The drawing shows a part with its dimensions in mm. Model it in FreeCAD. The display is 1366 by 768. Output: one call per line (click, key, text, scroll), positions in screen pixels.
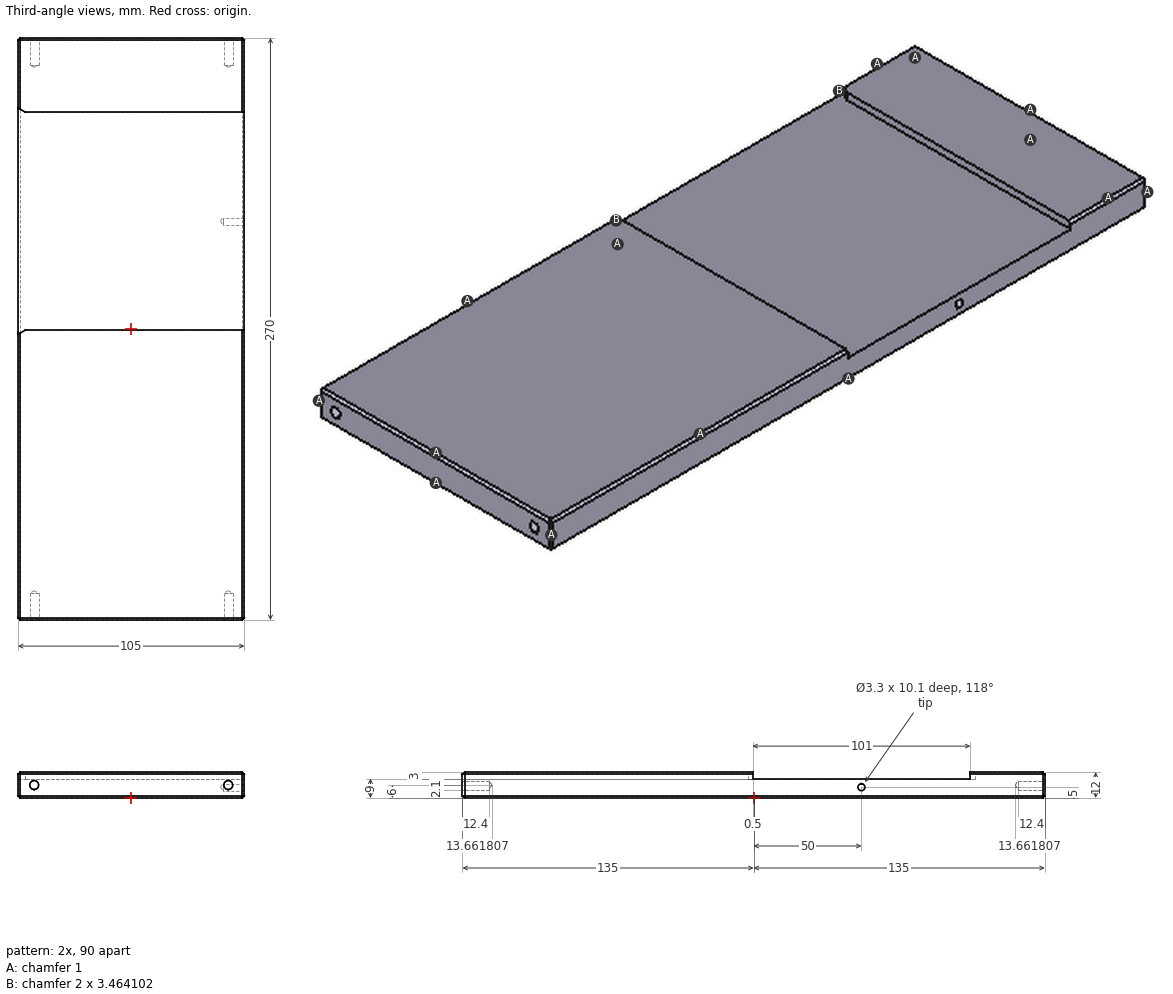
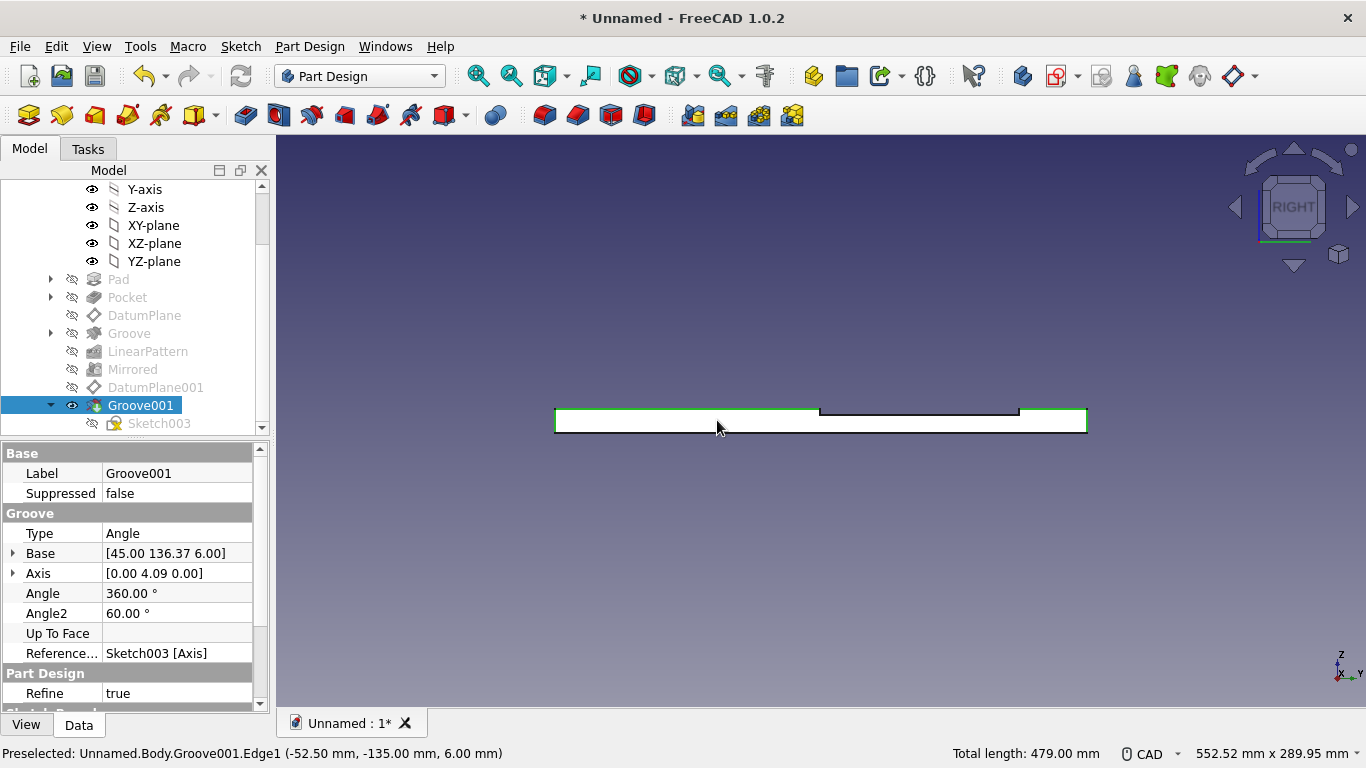
key(5)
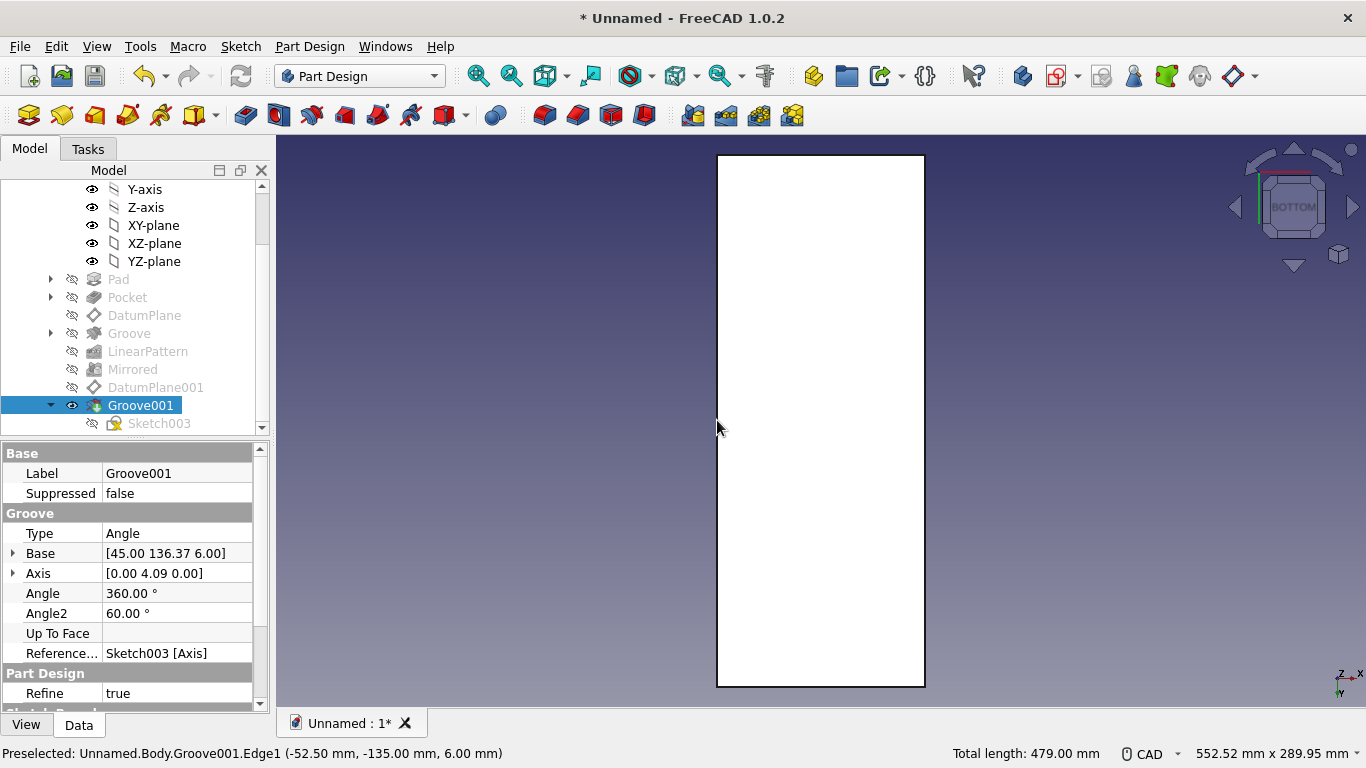
click(821, 572, ctrl)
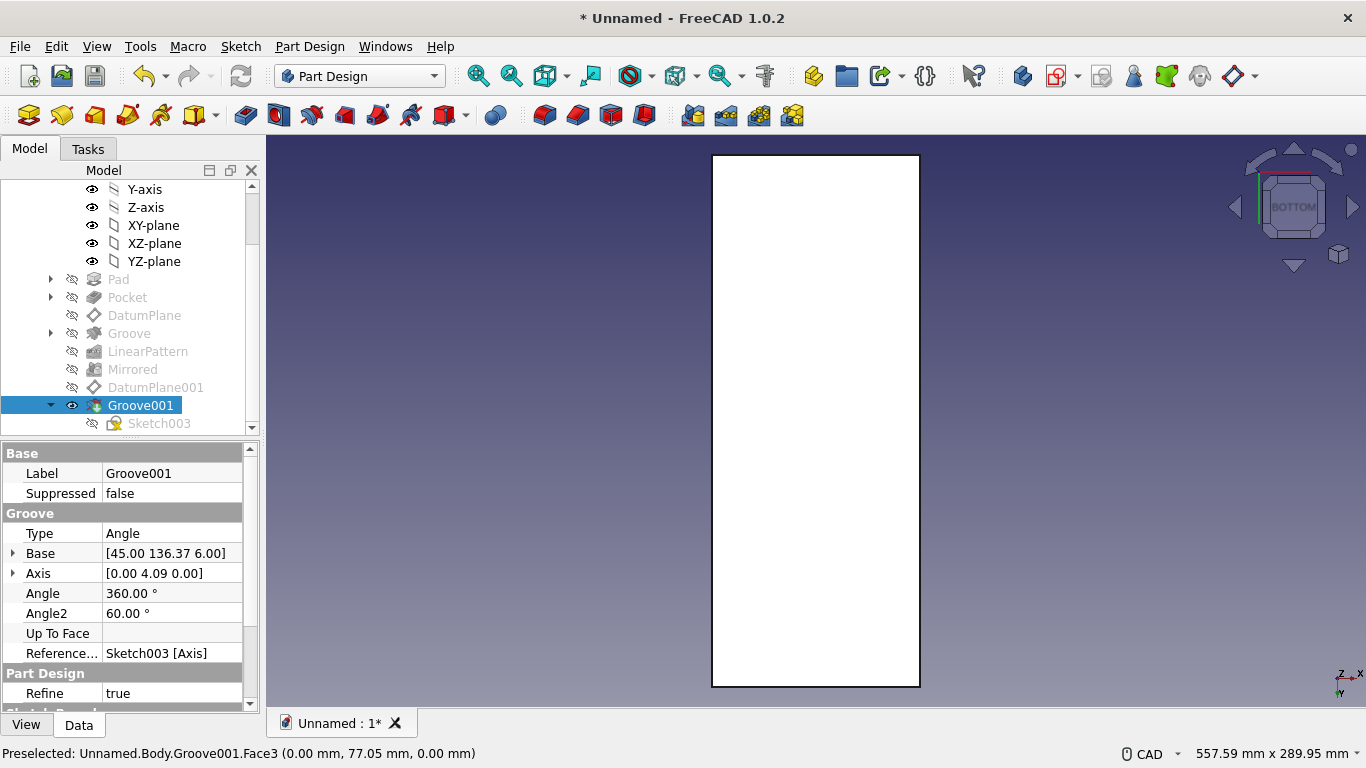
key(4)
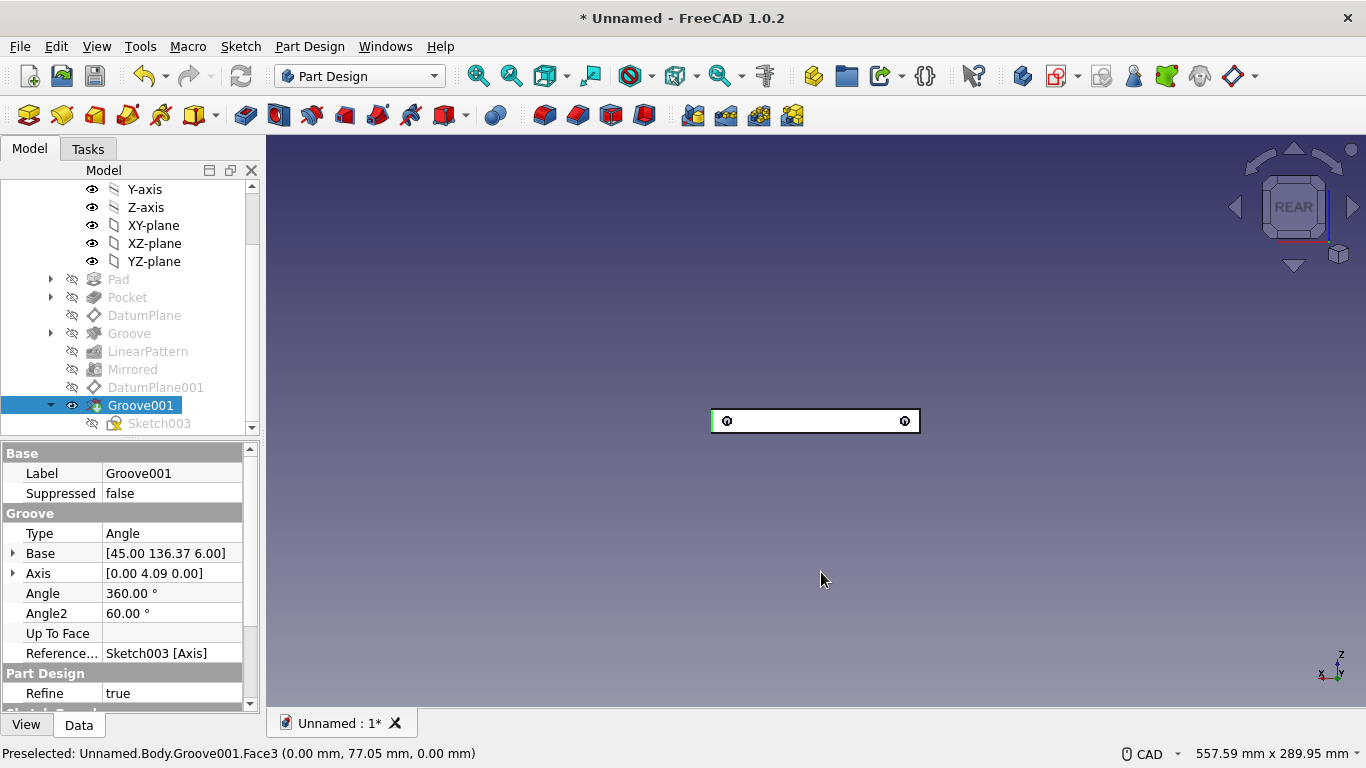
click(479, 76)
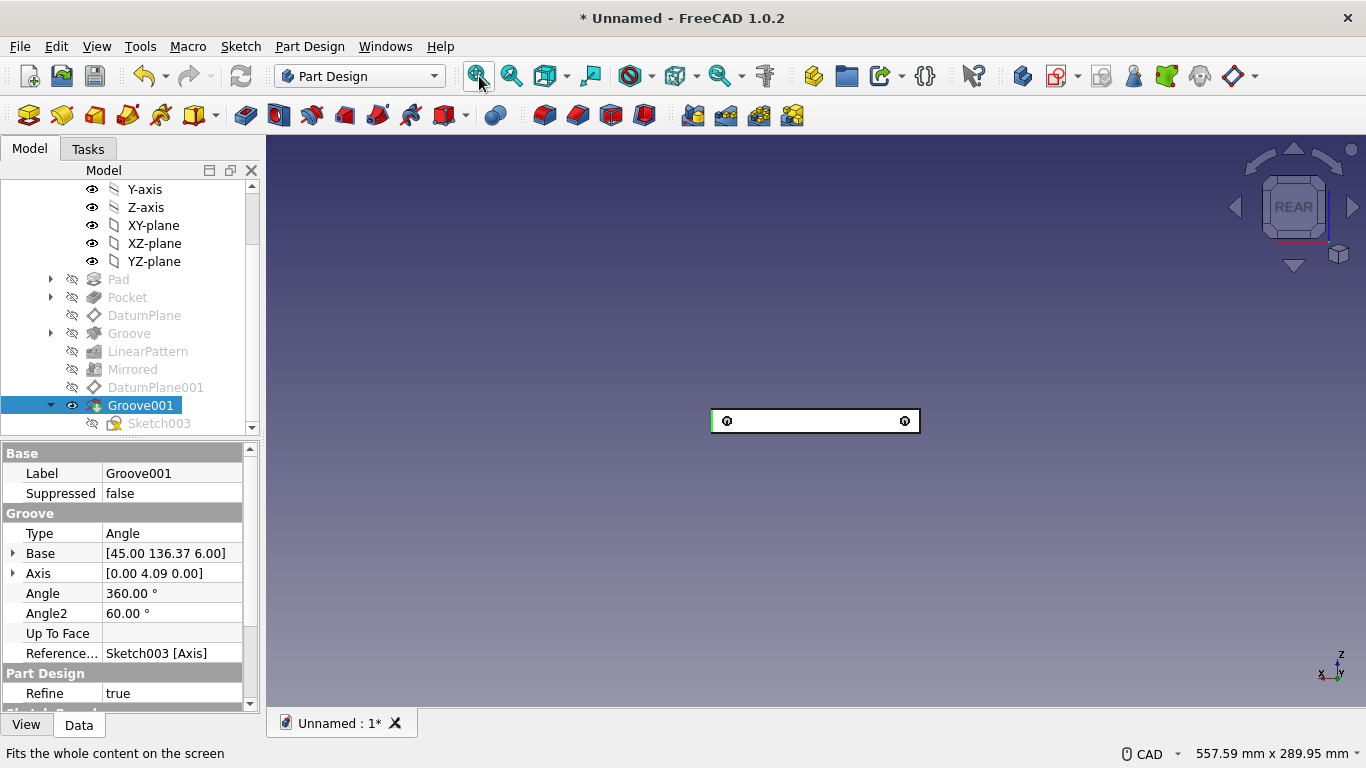
click(816, 408, ctrl)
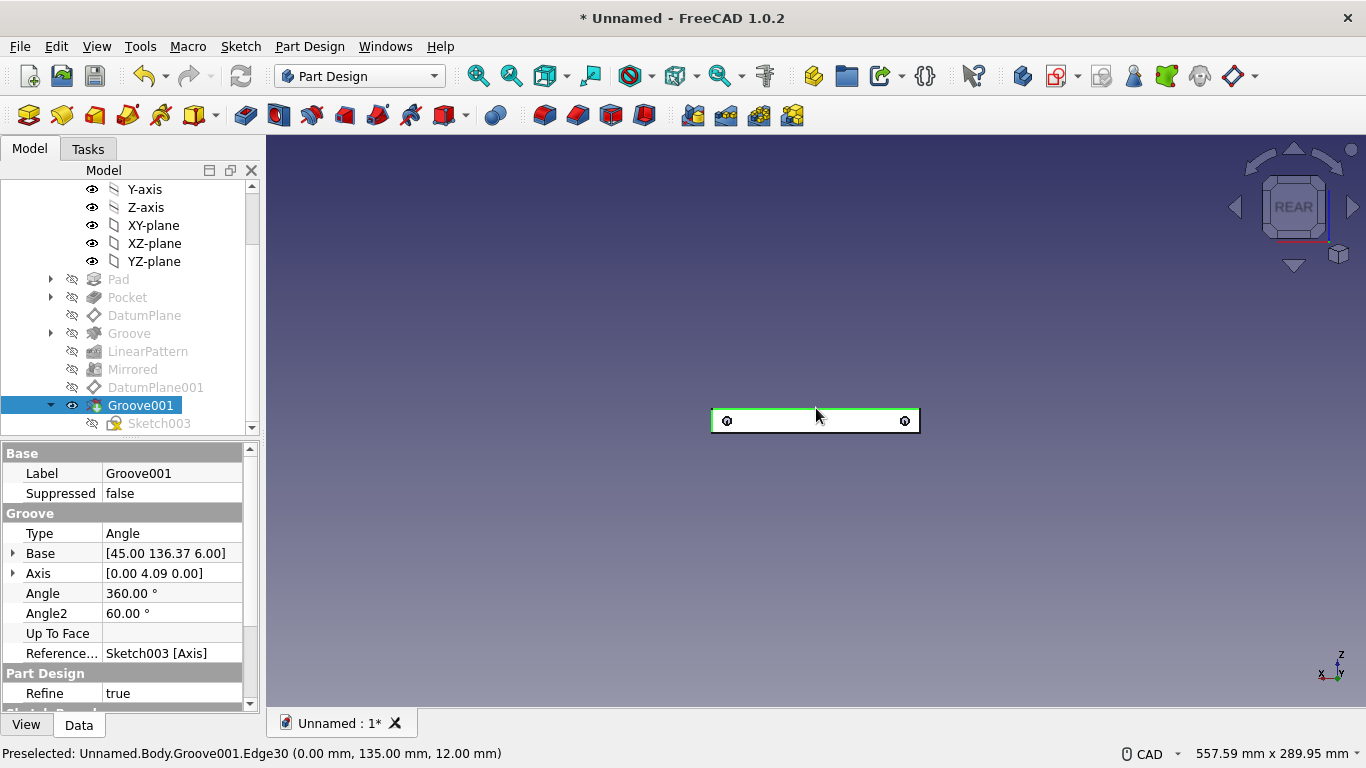
click(920, 420, ctrl)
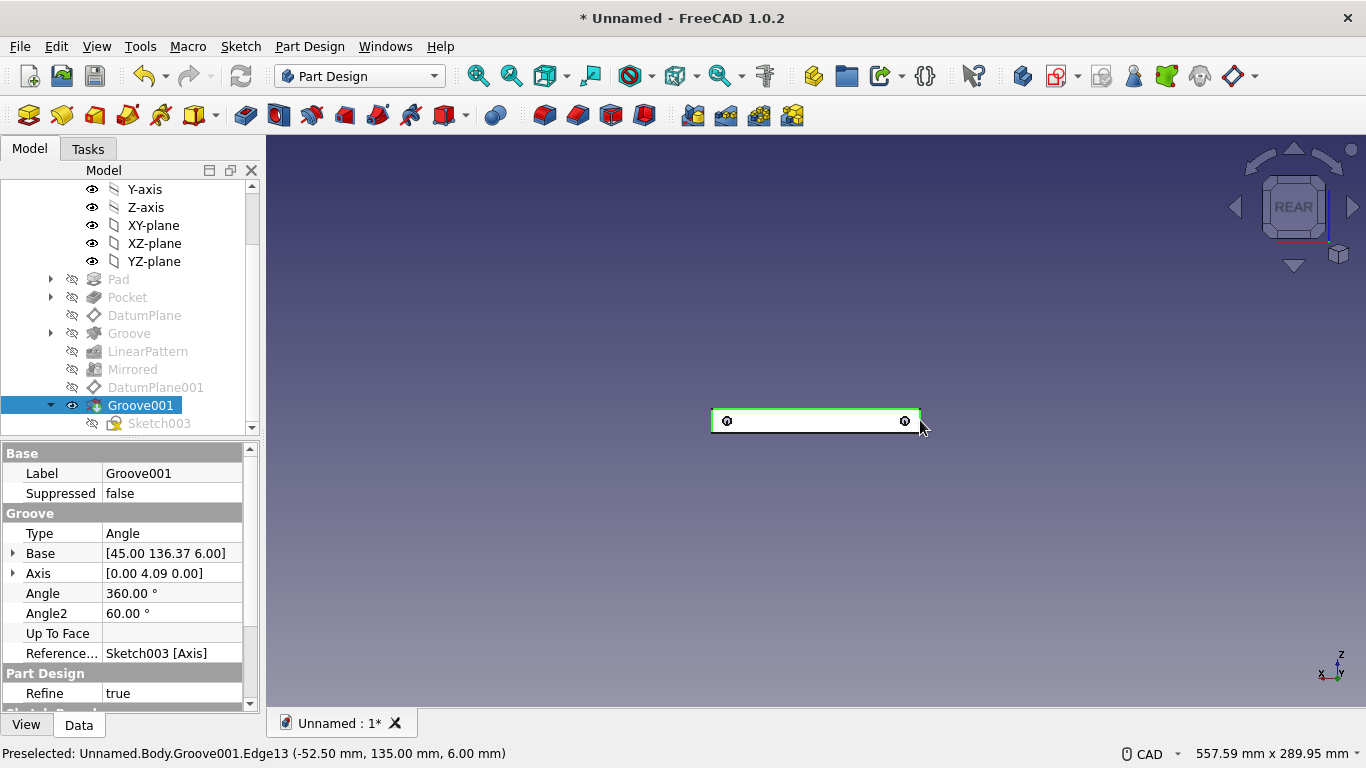
click(578, 116)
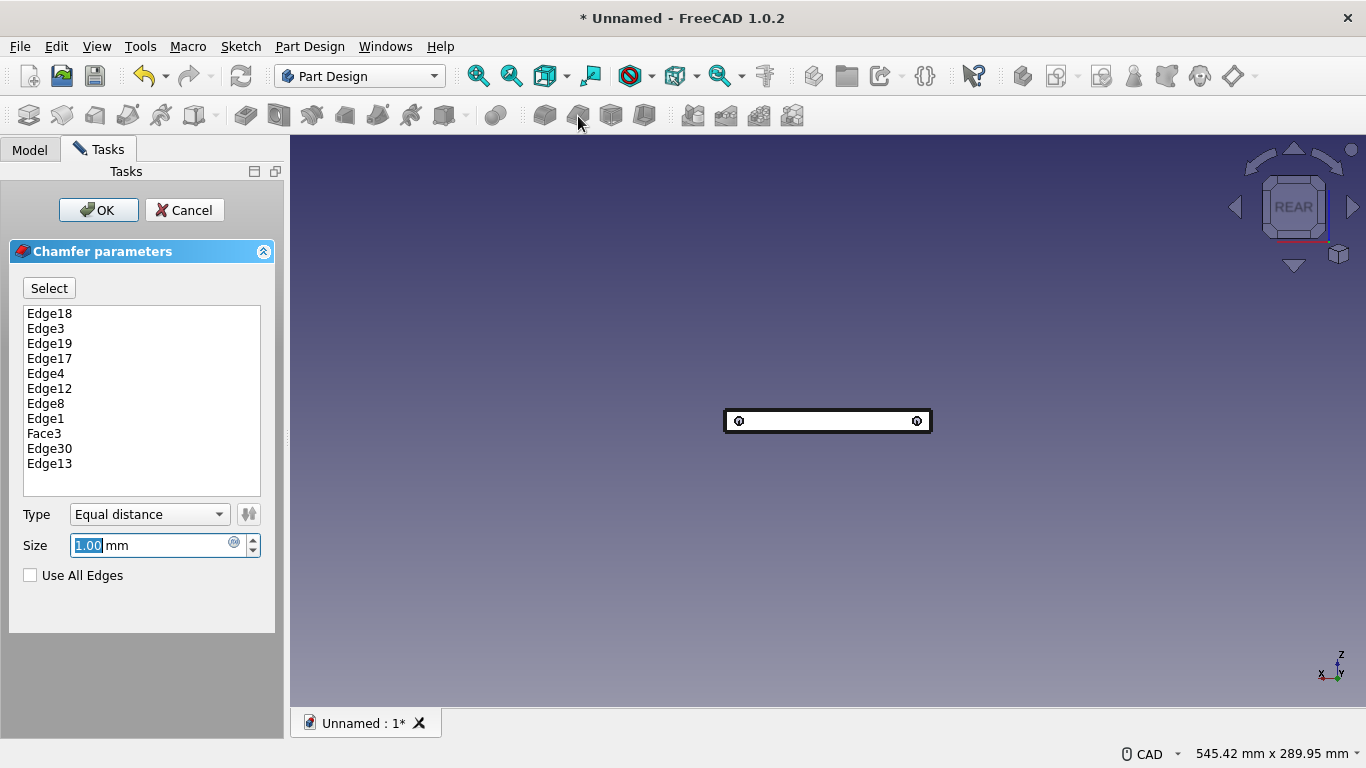
text(1)
key(Tab)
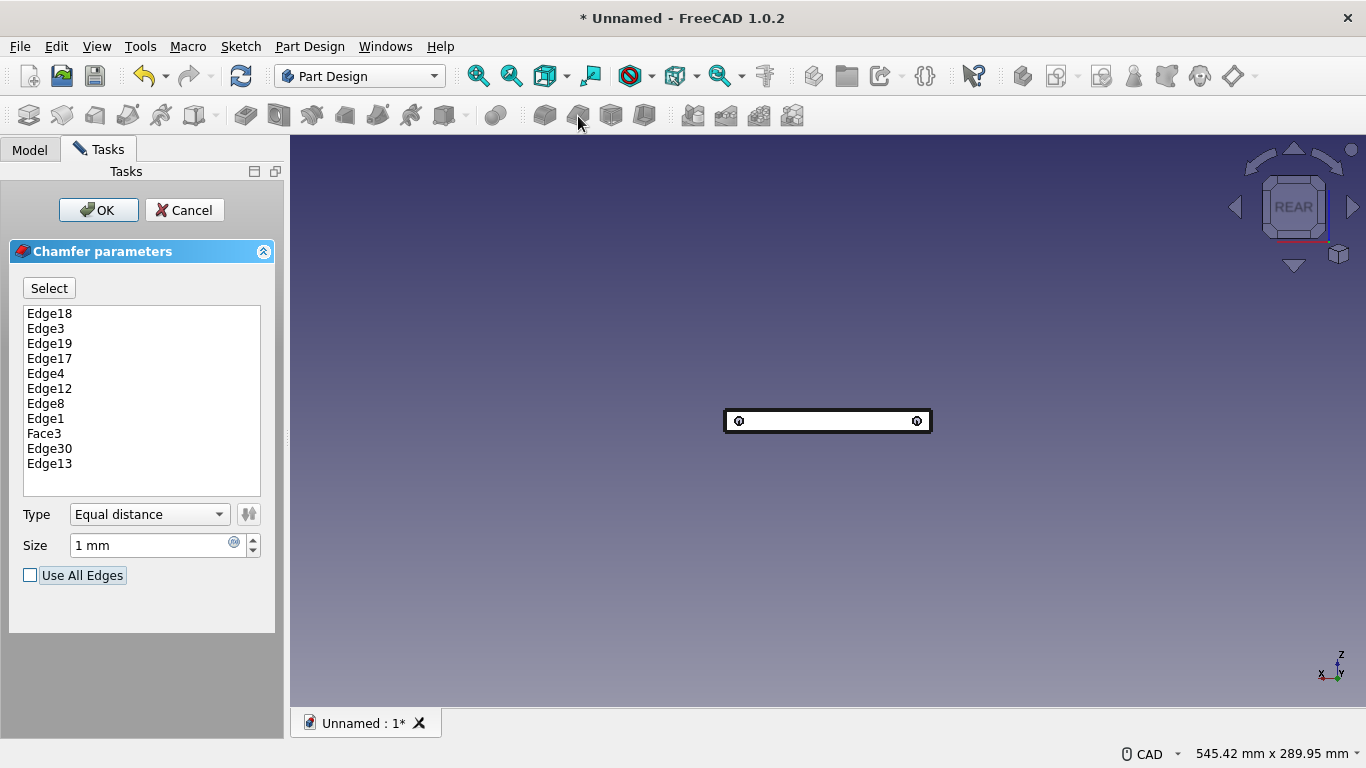
click(99, 210)